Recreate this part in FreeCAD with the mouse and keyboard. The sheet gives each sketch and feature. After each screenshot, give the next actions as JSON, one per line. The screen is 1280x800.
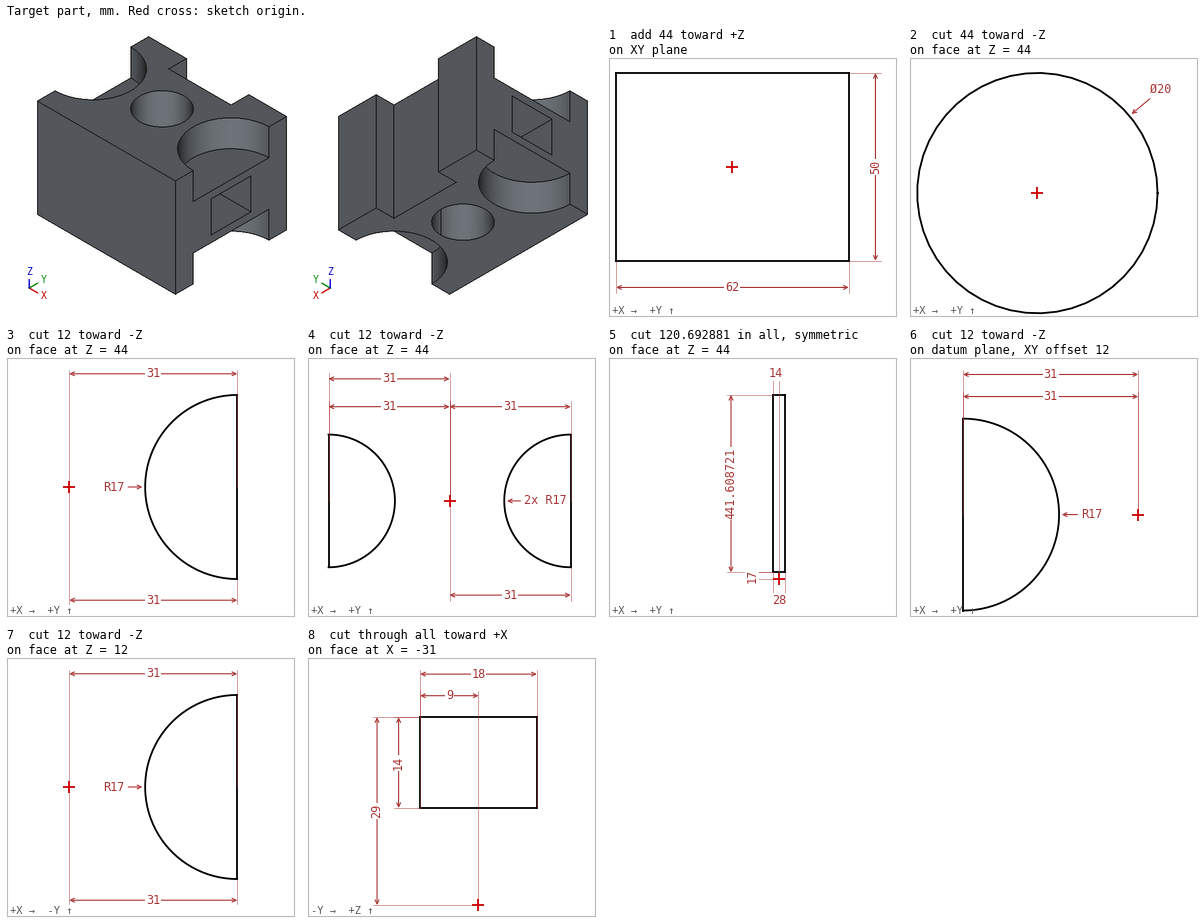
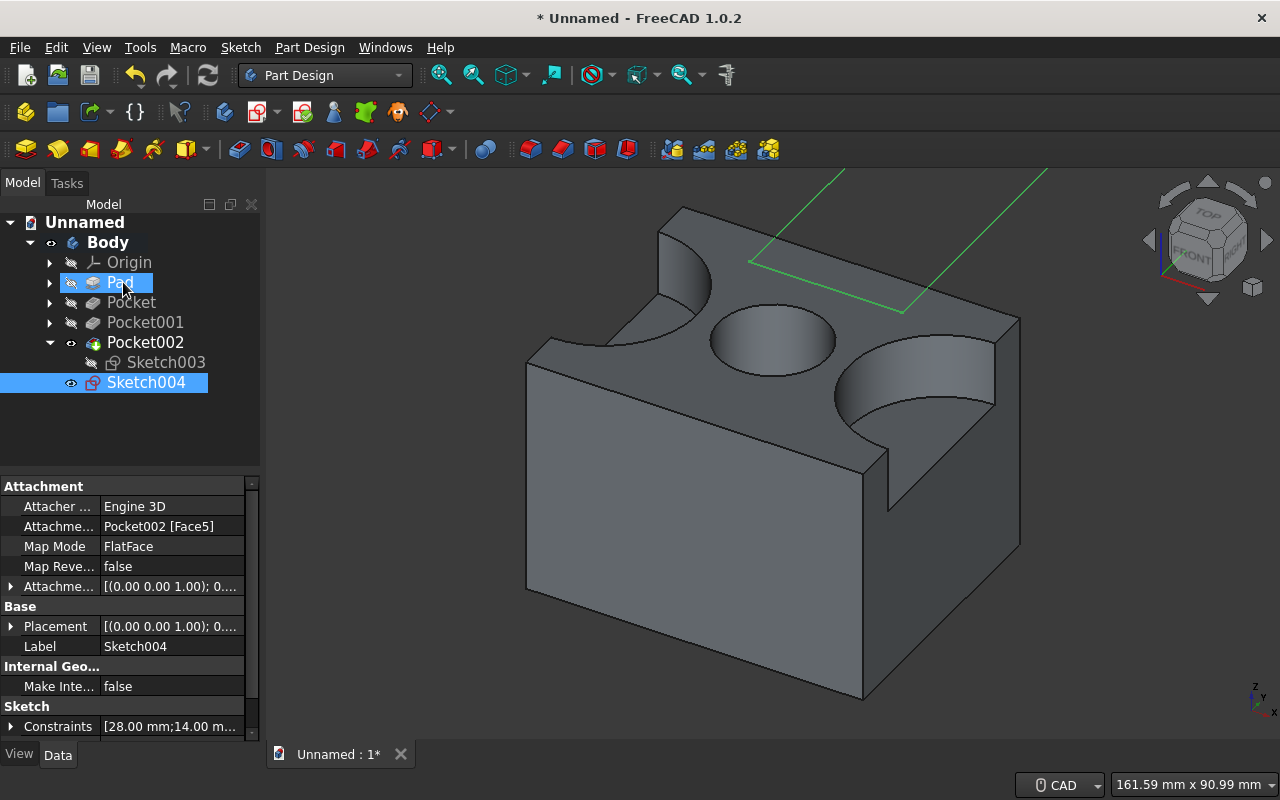
{"action": "left_click", "coordinate": [240, 150]}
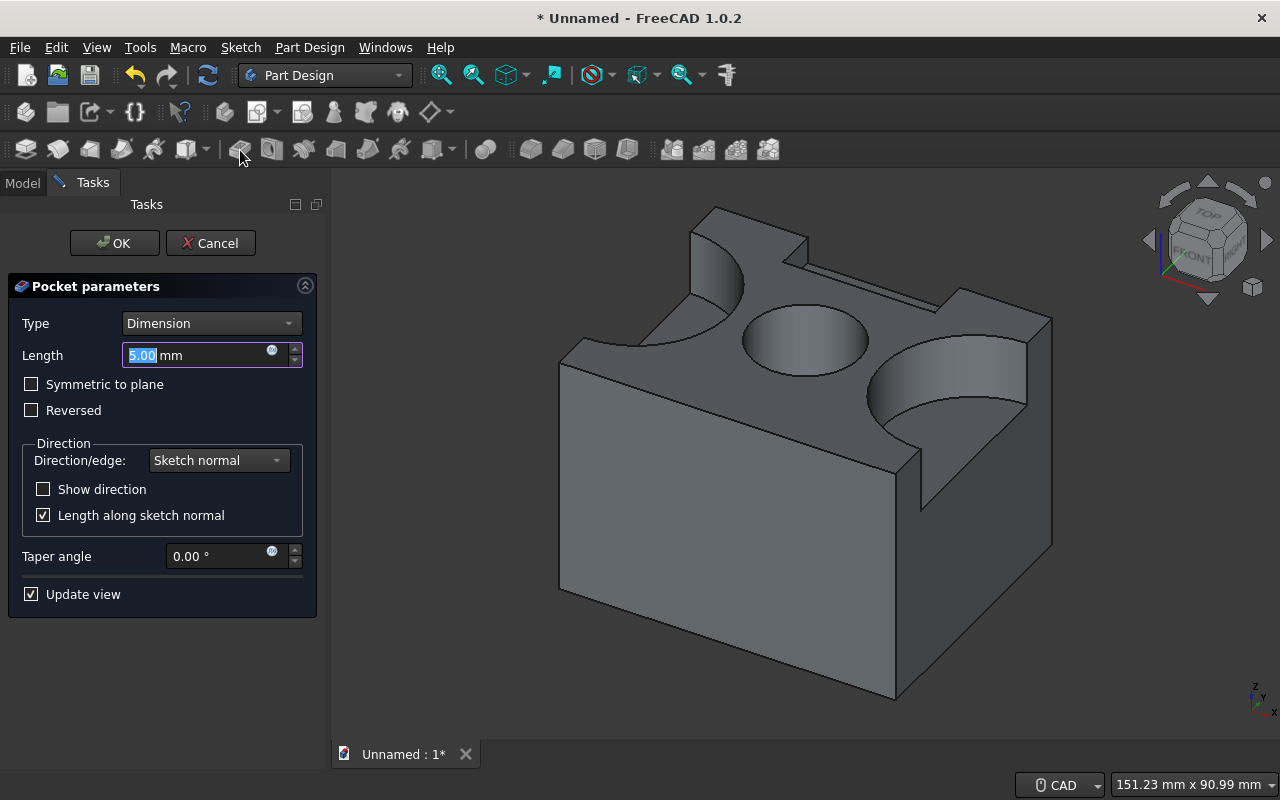
{"action": "type", "text": "120.692881"}
{"action": "key", "text": "Tab"}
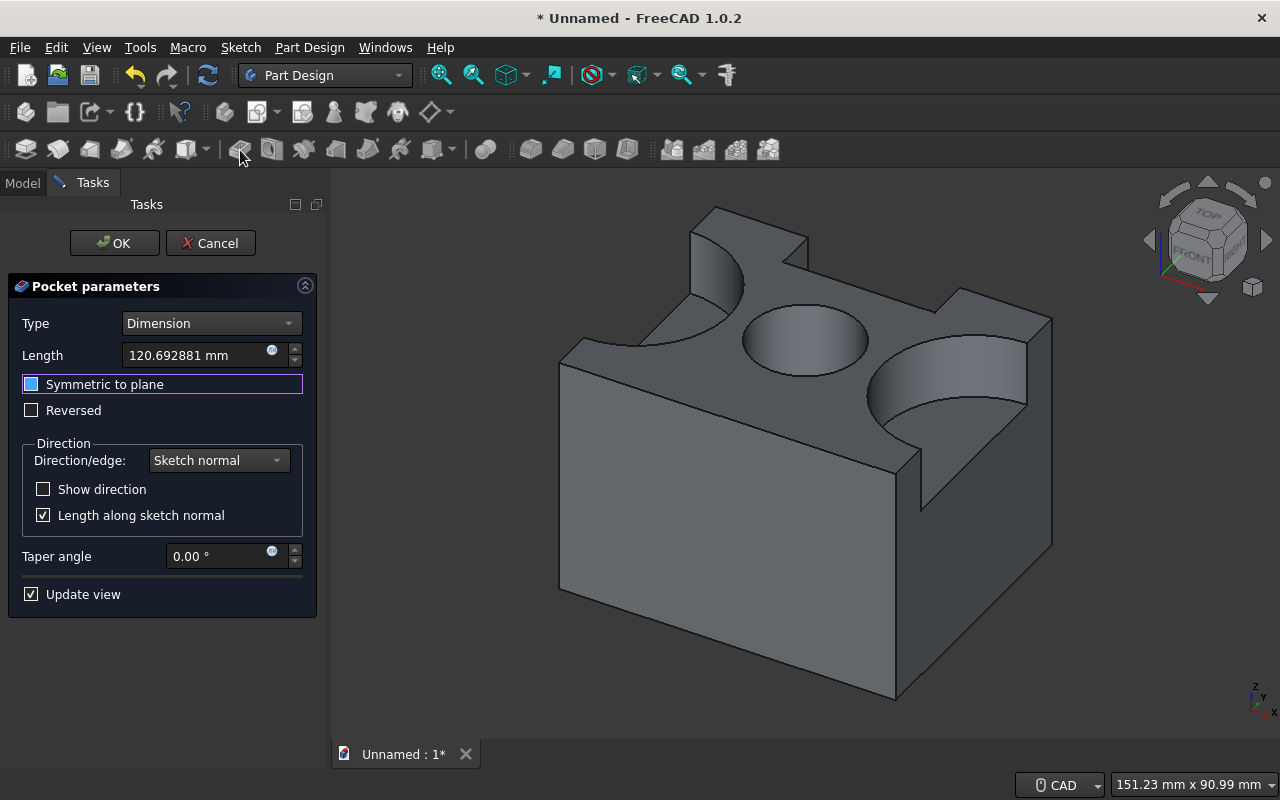
{"action": "left_click", "coordinate": [30, 384]}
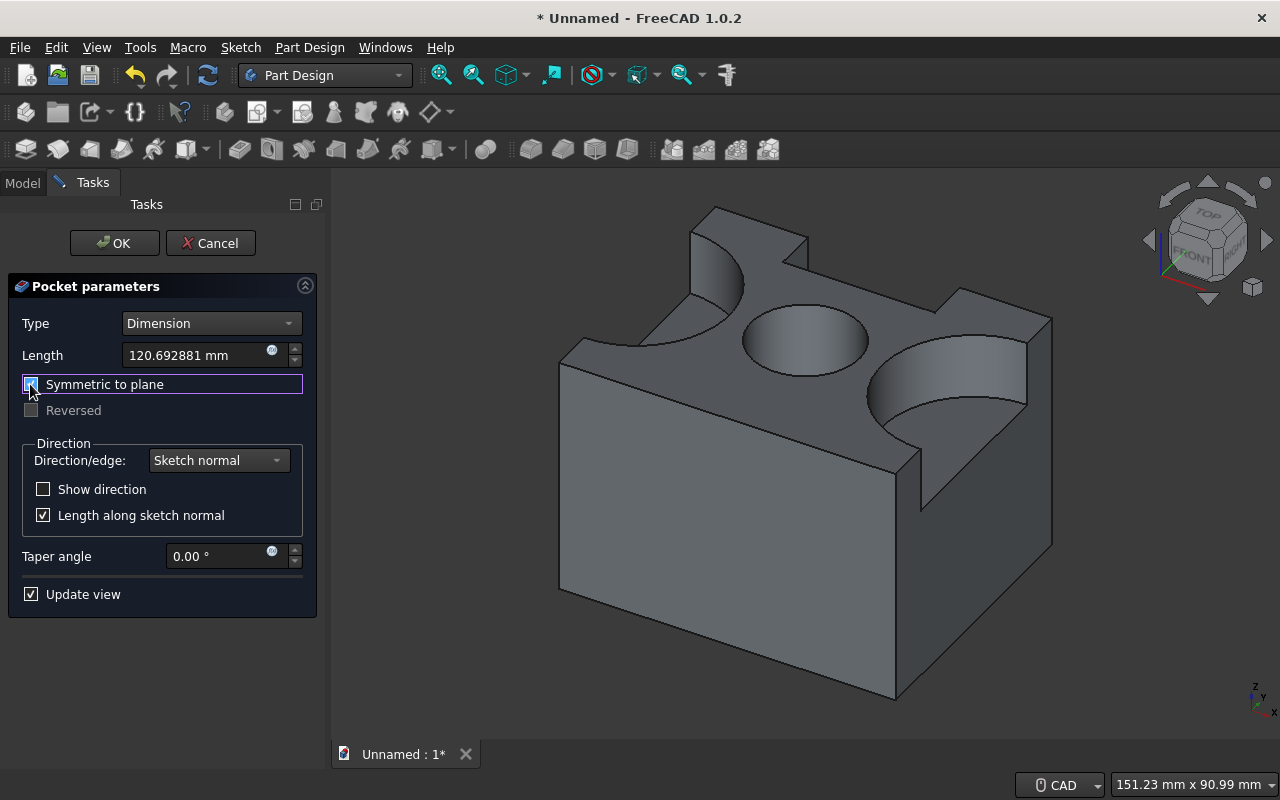
{"action": "left_click", "coordinate": [115, 243]}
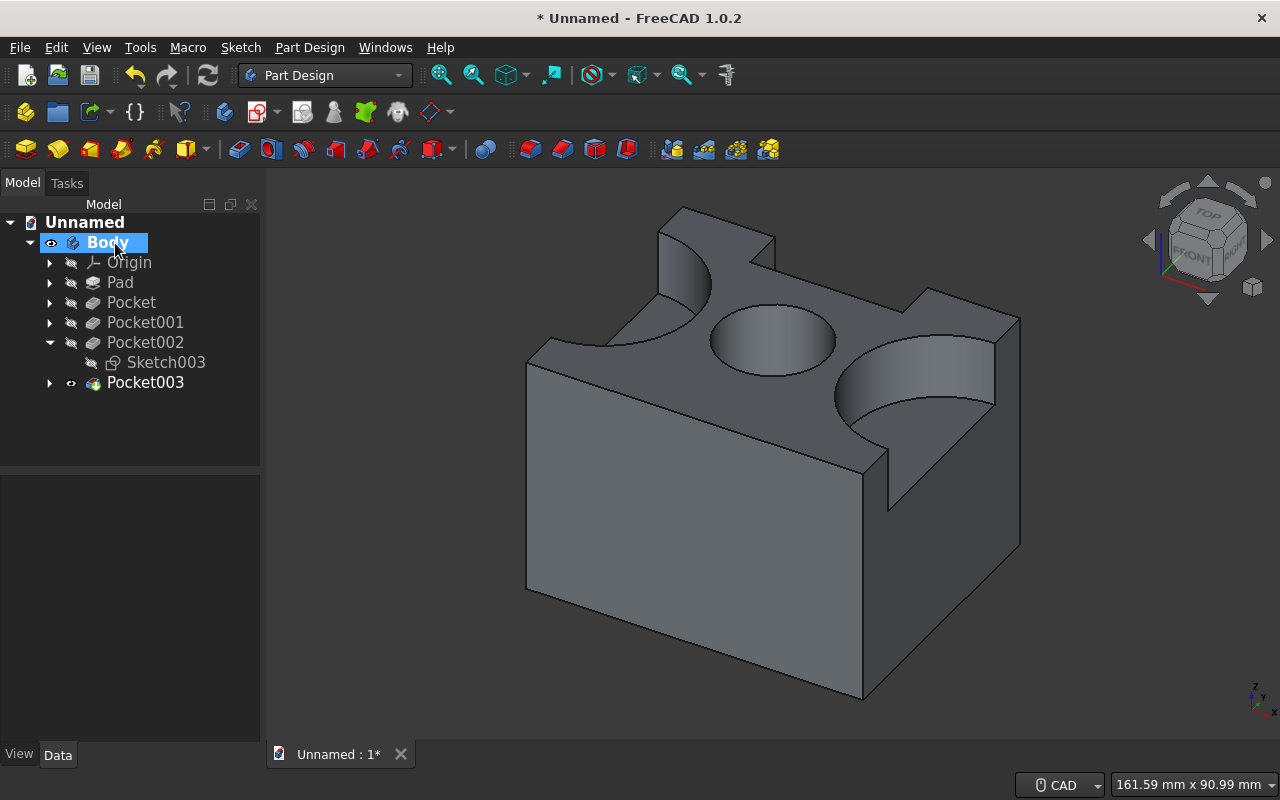
{"action": "left_click", "coordinate": [50, 263]}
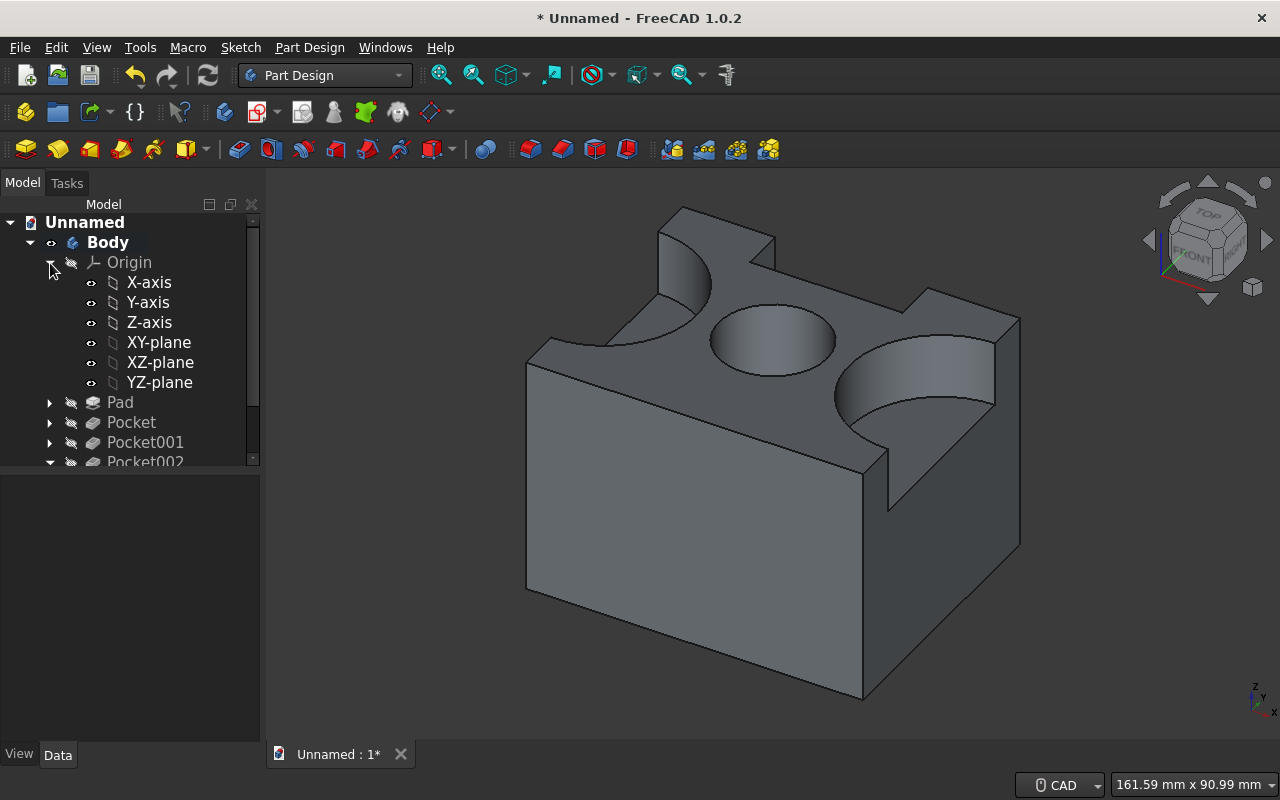
{"action": "left_click", "coordinate": [136, 343]}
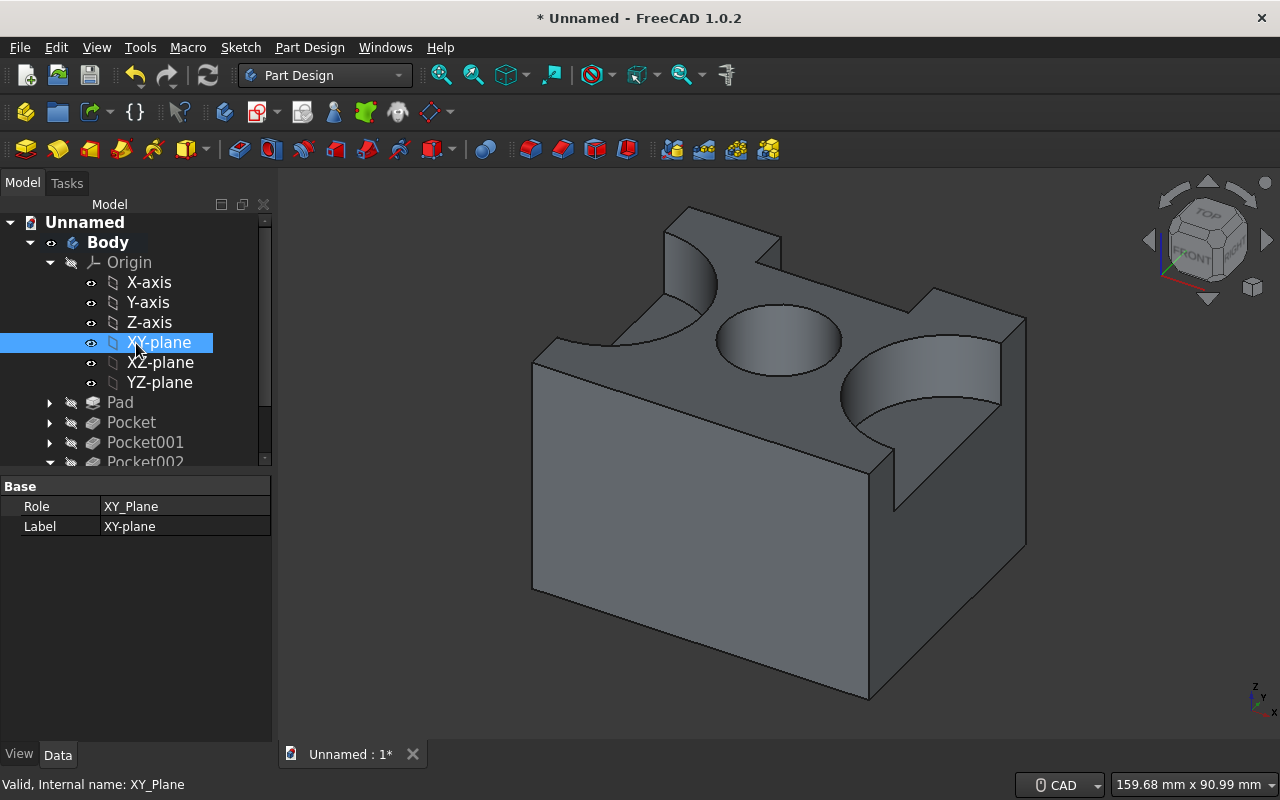
{"action": "left_click", "coordinate": [430, 112]}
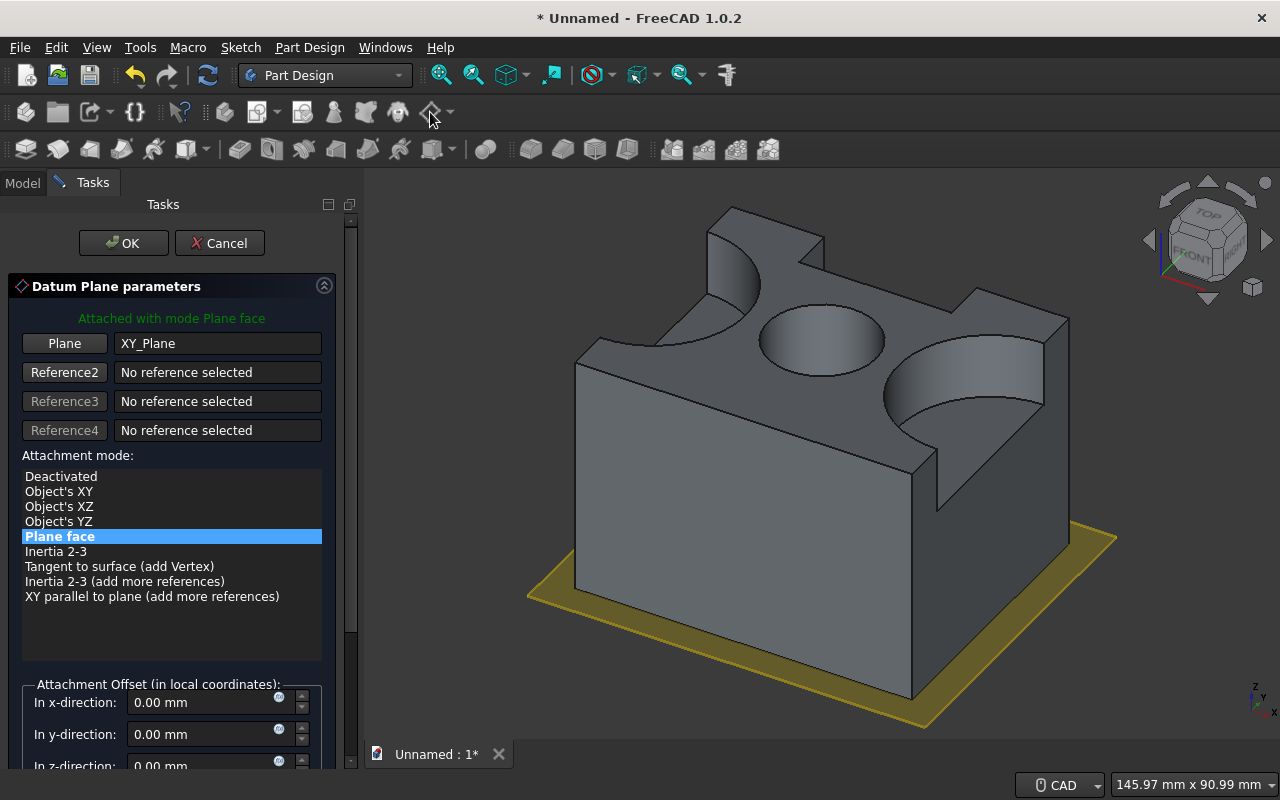
{"action": "scroll", "coordinate": [351, 491], "scroll_direction": "down", "scroll_amount": 2}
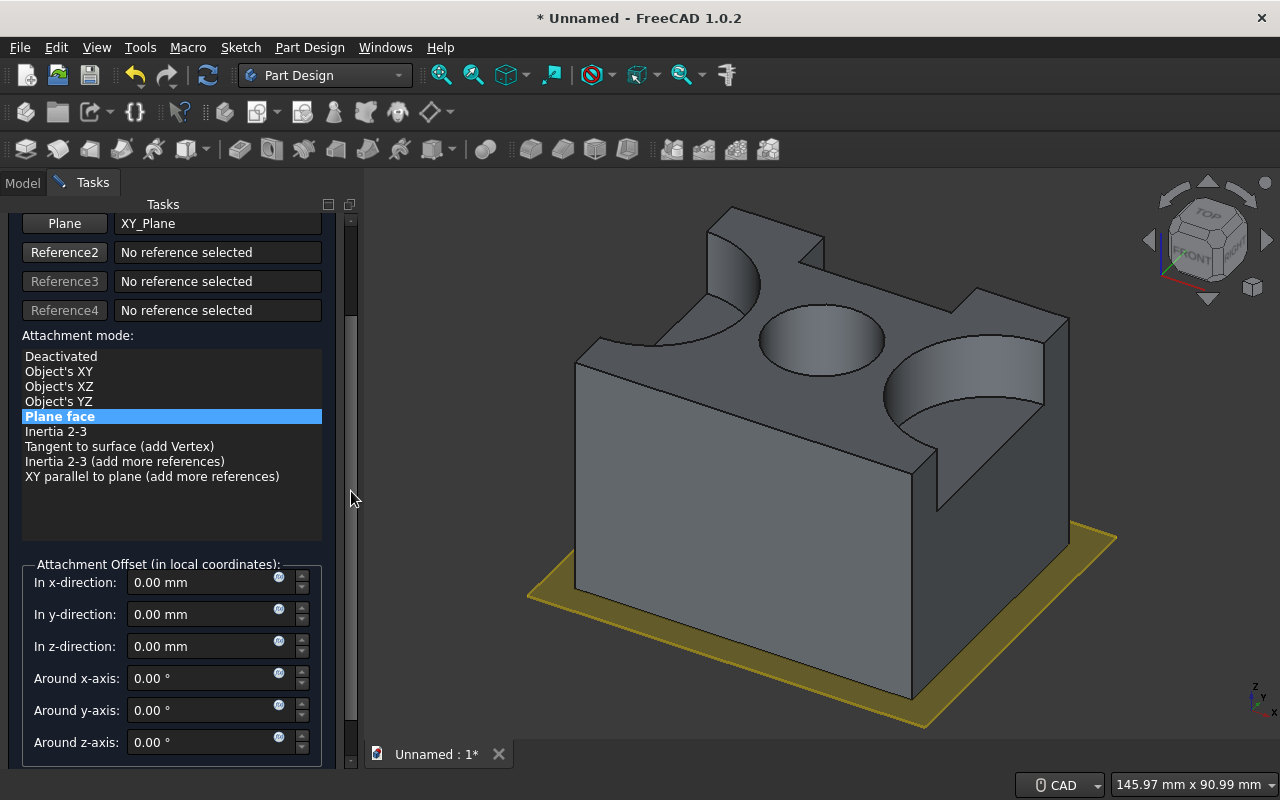
{"action": "triple_click", "coordinate": [210, 646]}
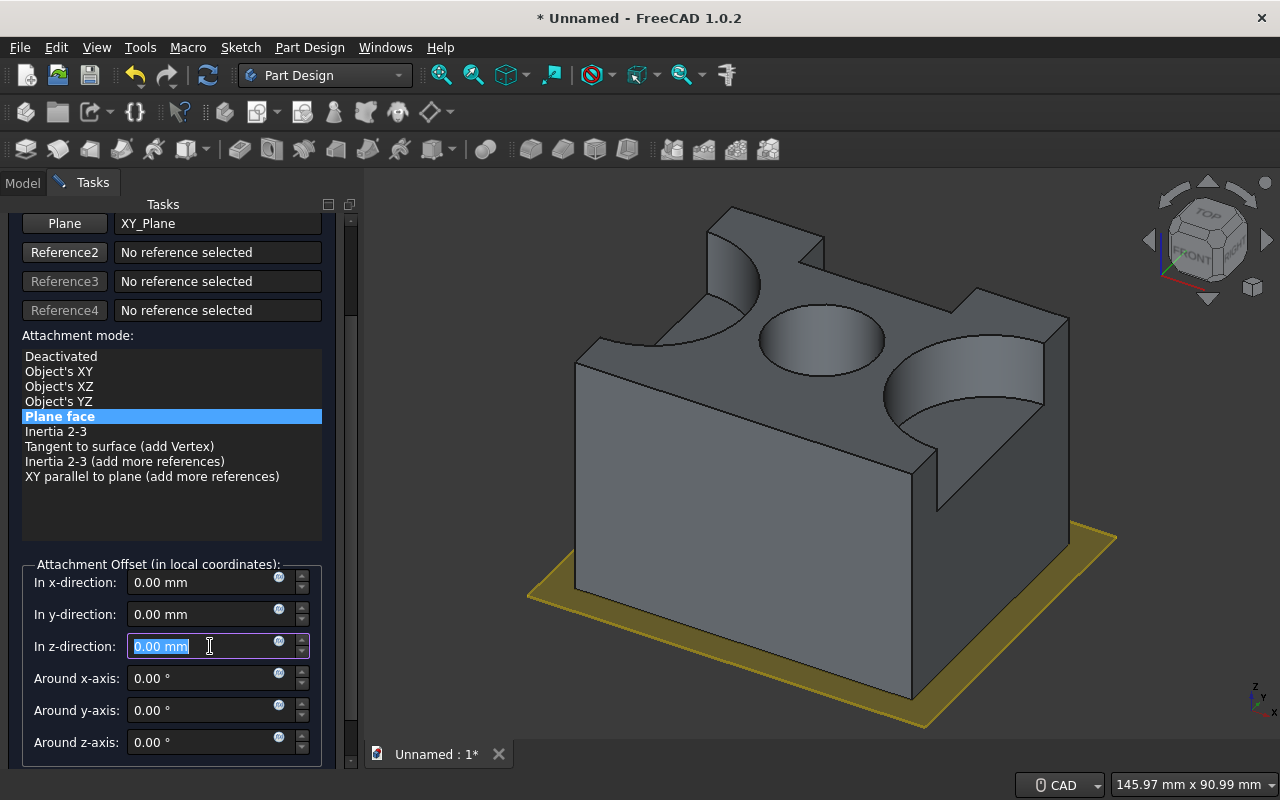
{"action": "type", "text": "12"}
{"action": "key", "text": "Tab"}